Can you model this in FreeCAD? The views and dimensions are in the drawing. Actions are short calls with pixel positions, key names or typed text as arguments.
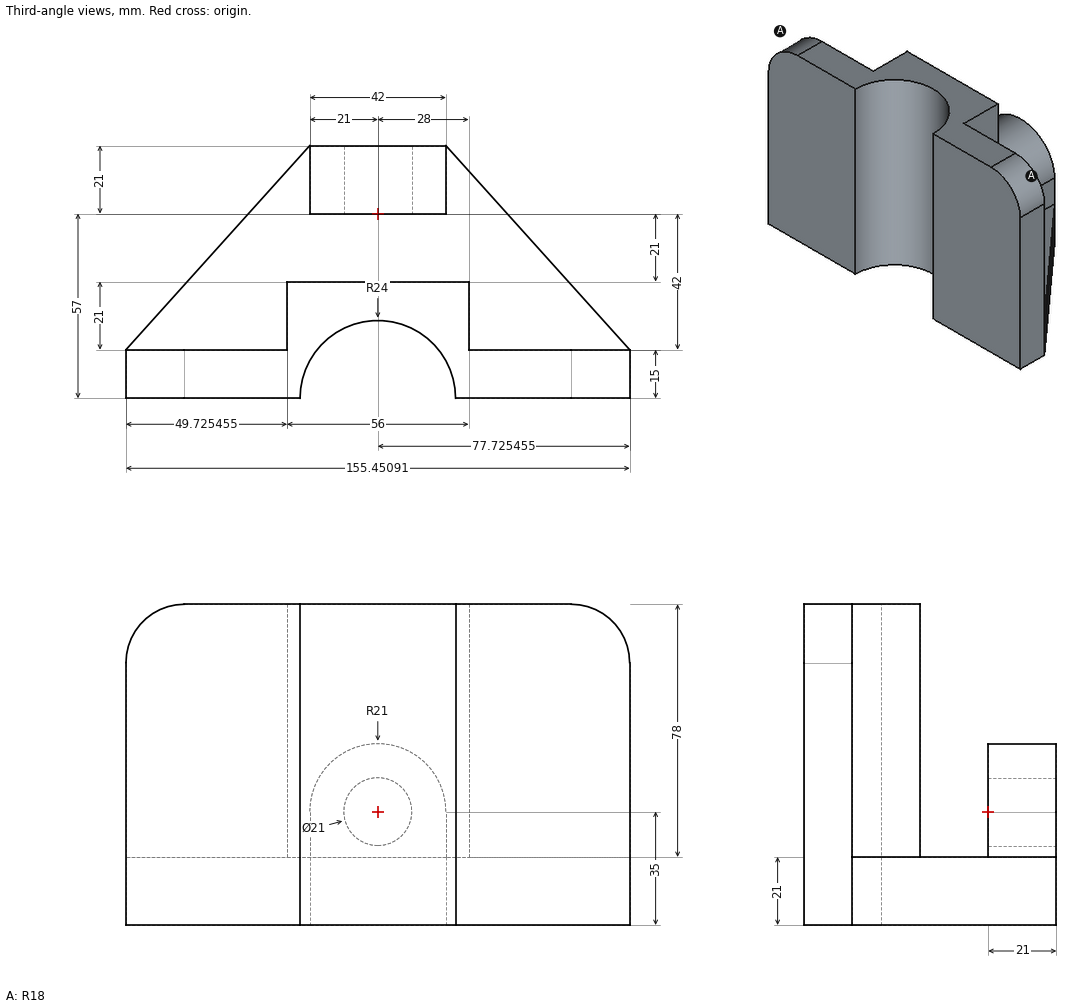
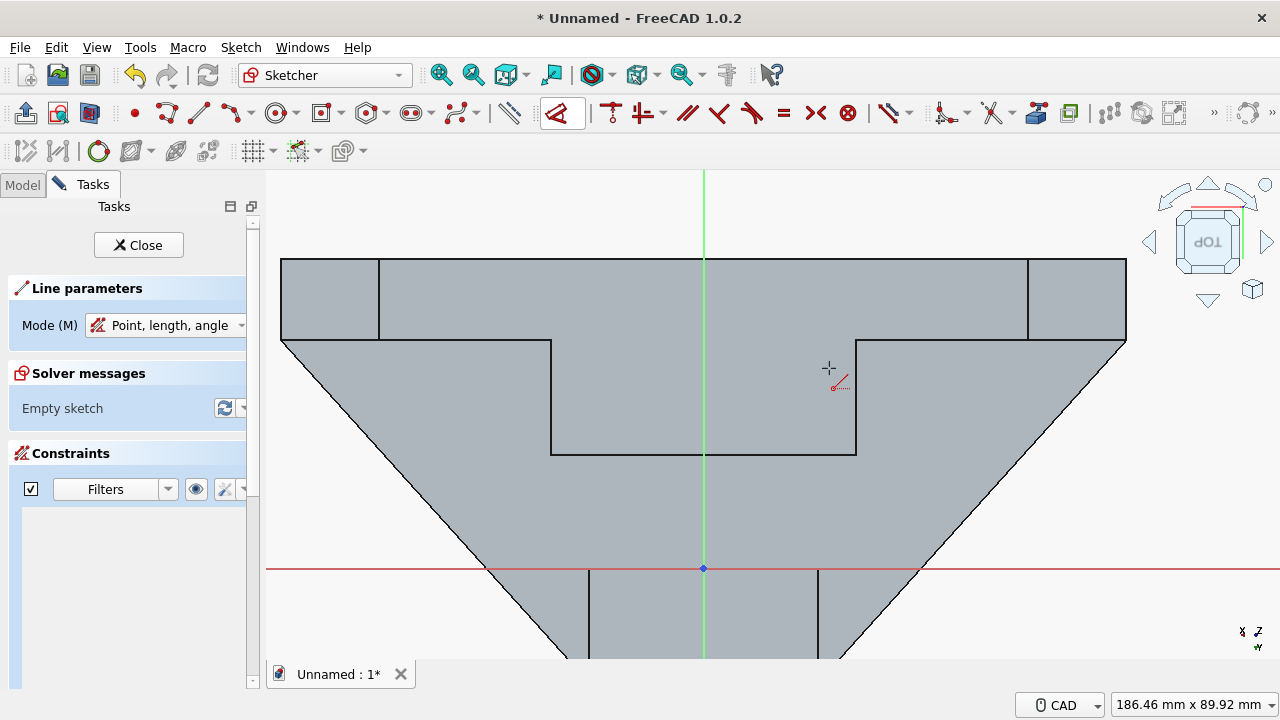
click(834, 259)
click(573, 259)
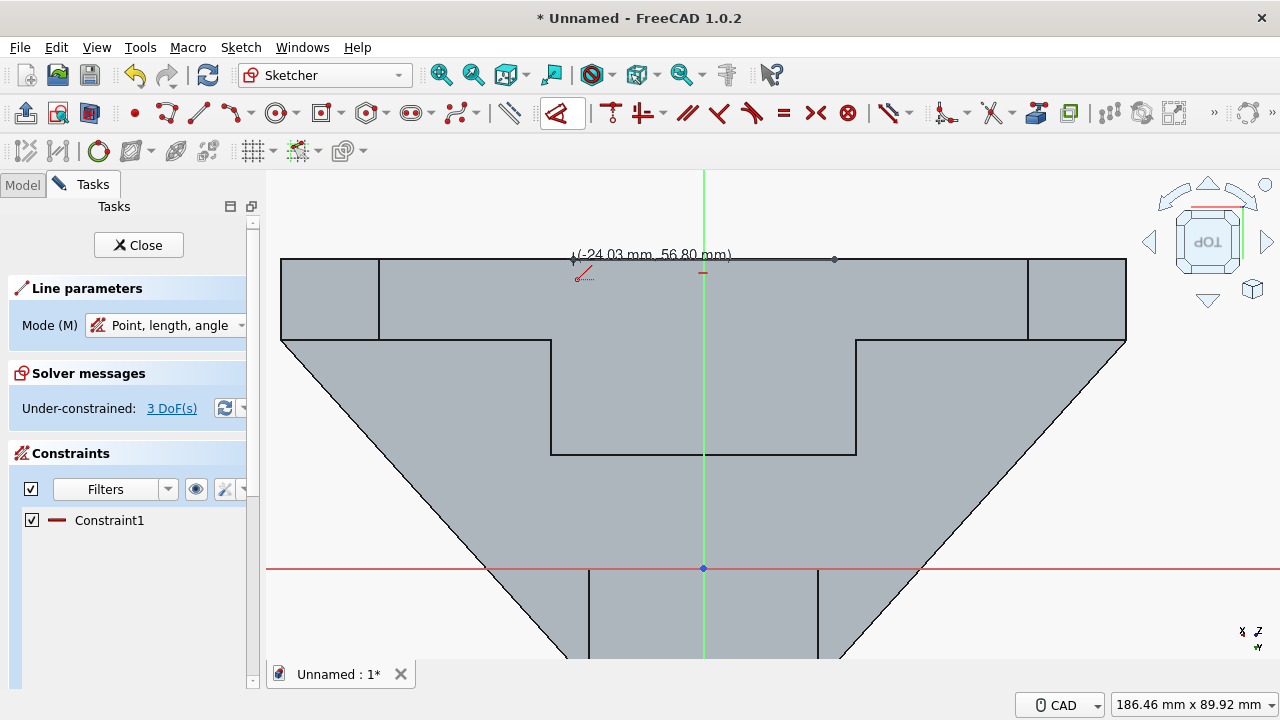
click(232, 114)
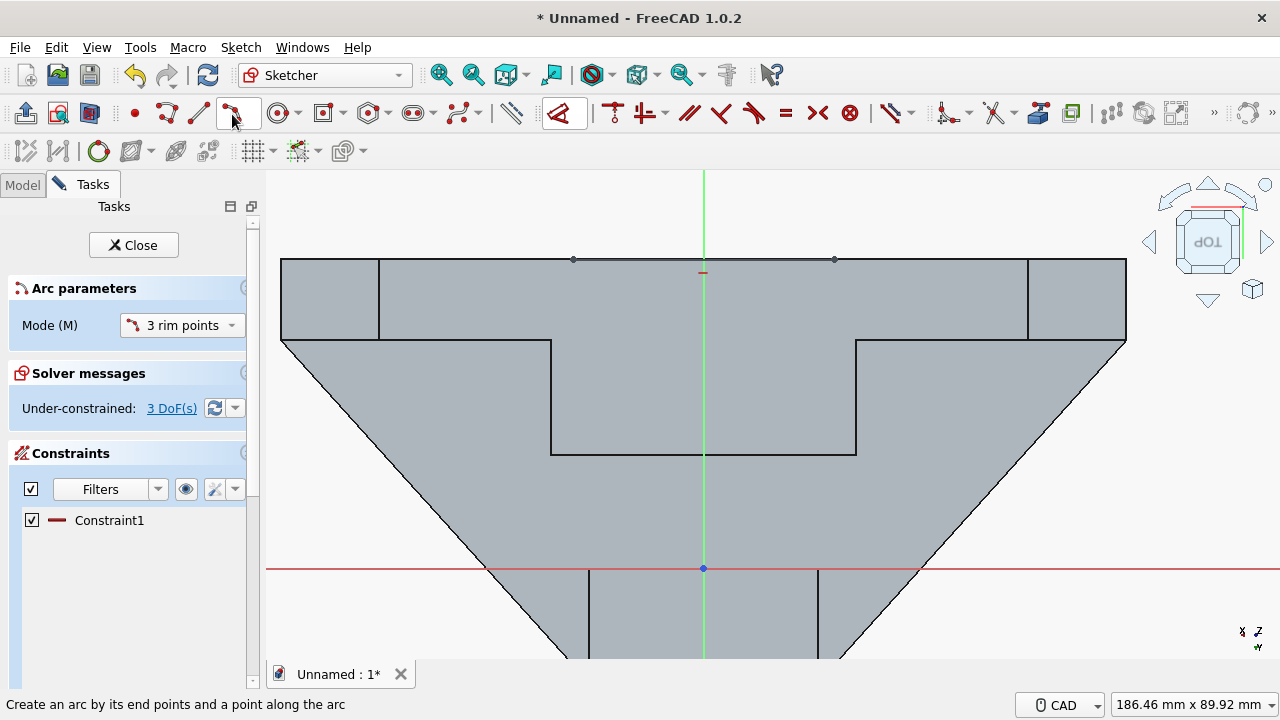
click(573, 260)
click(834, 260)
click(663, 383)
key(Escape)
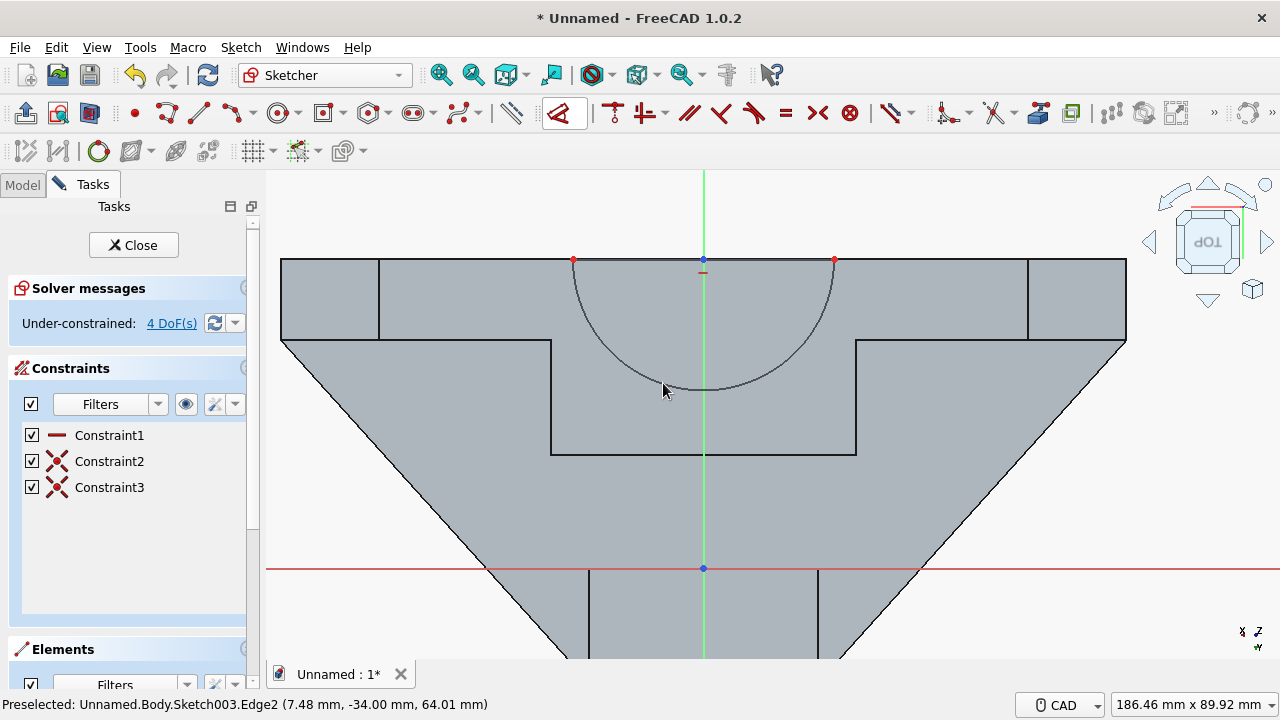
click(704, 260)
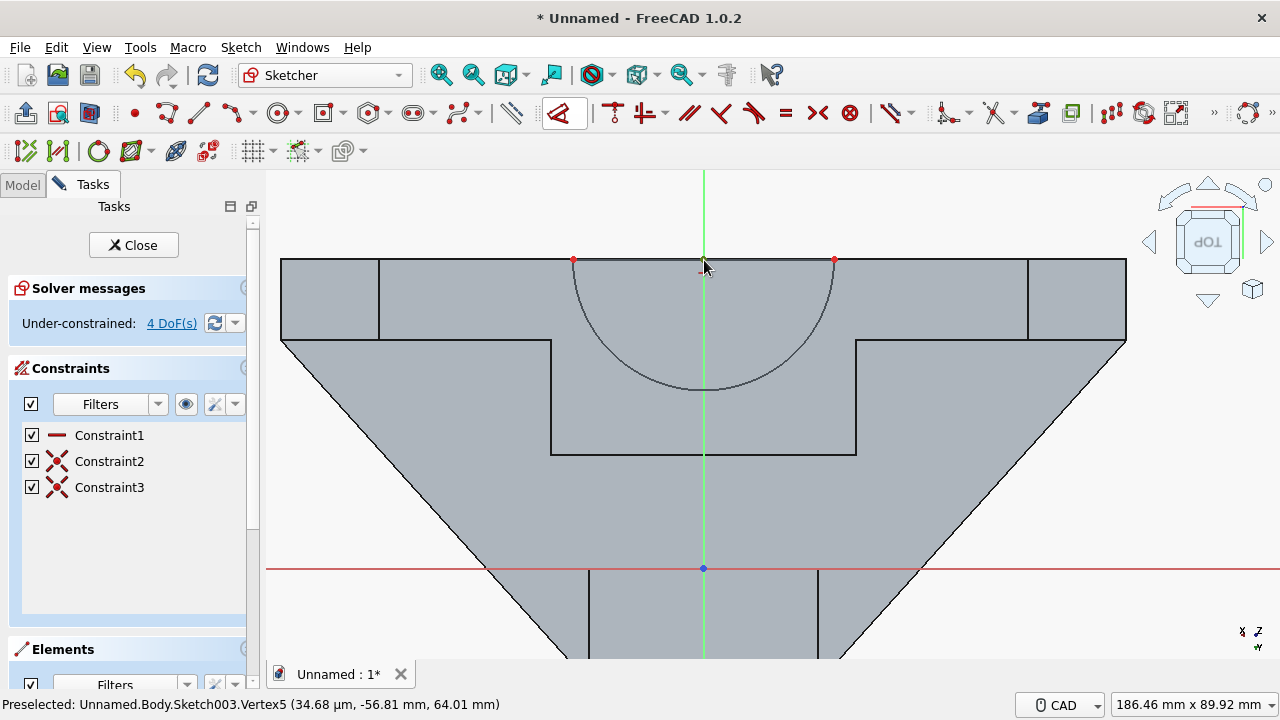
click(704, 600)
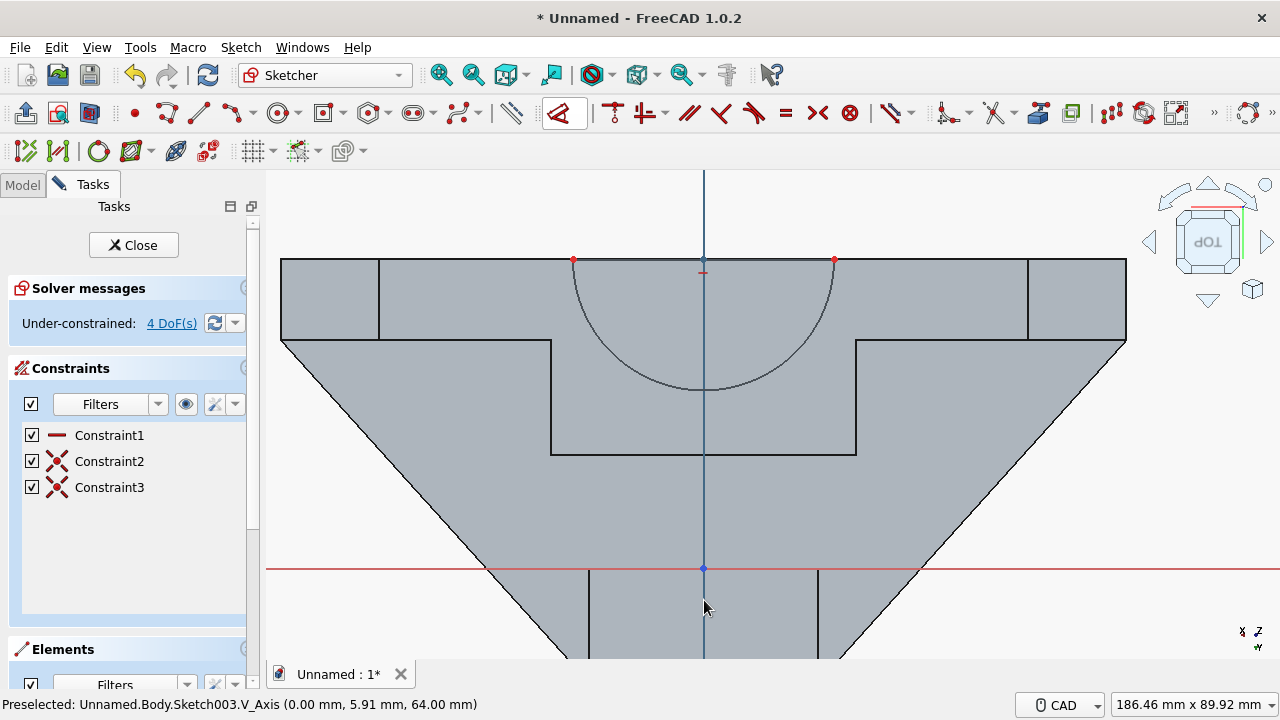
click(614, 114)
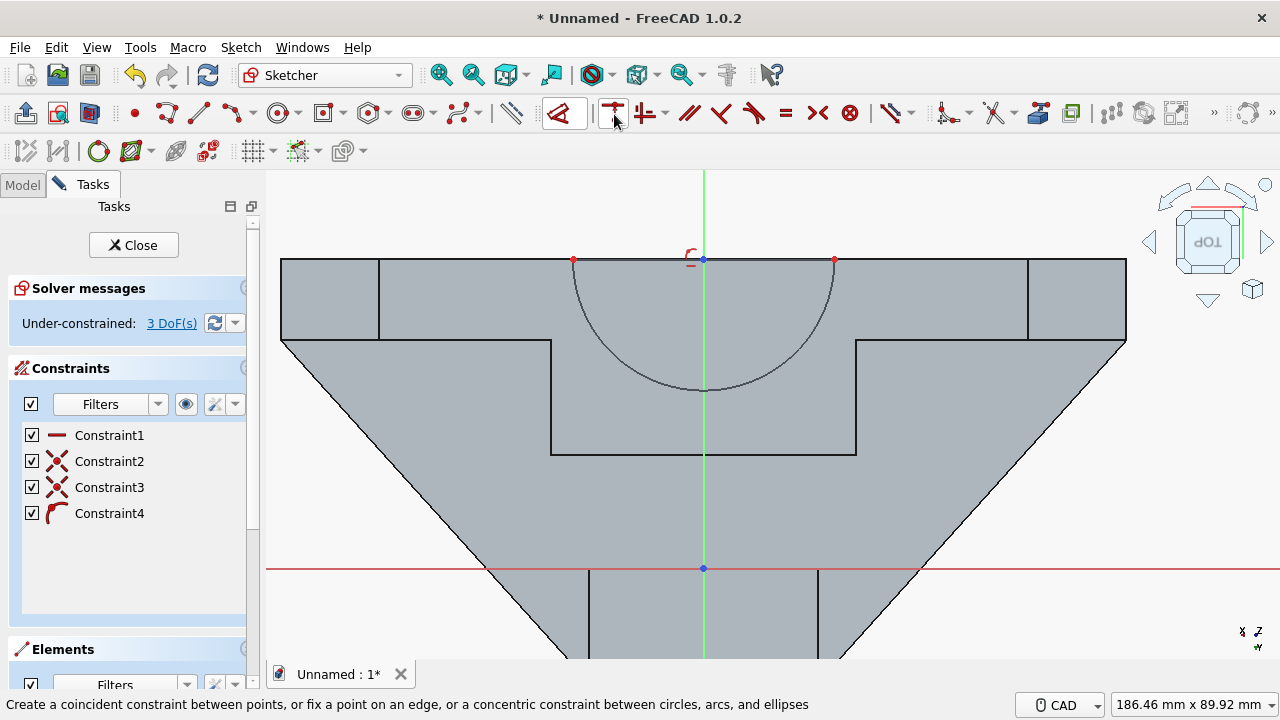
click(627, 366)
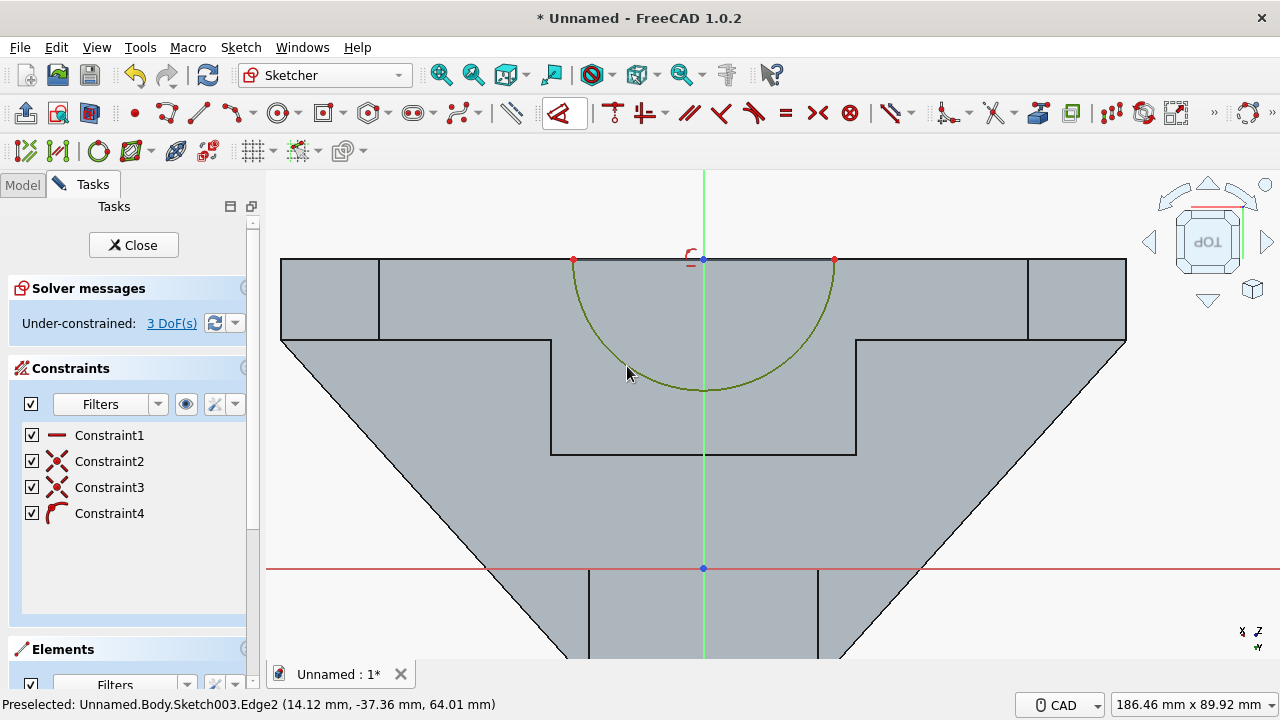
click(582, 114)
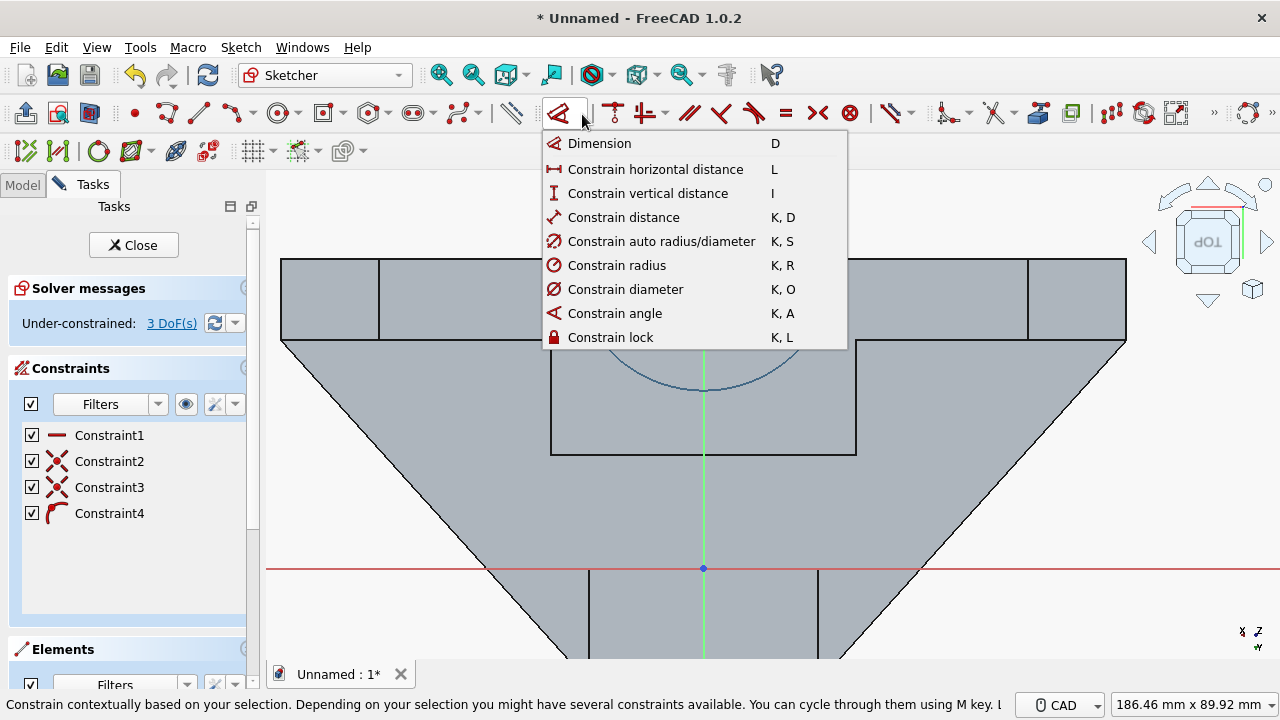
click(695, 265)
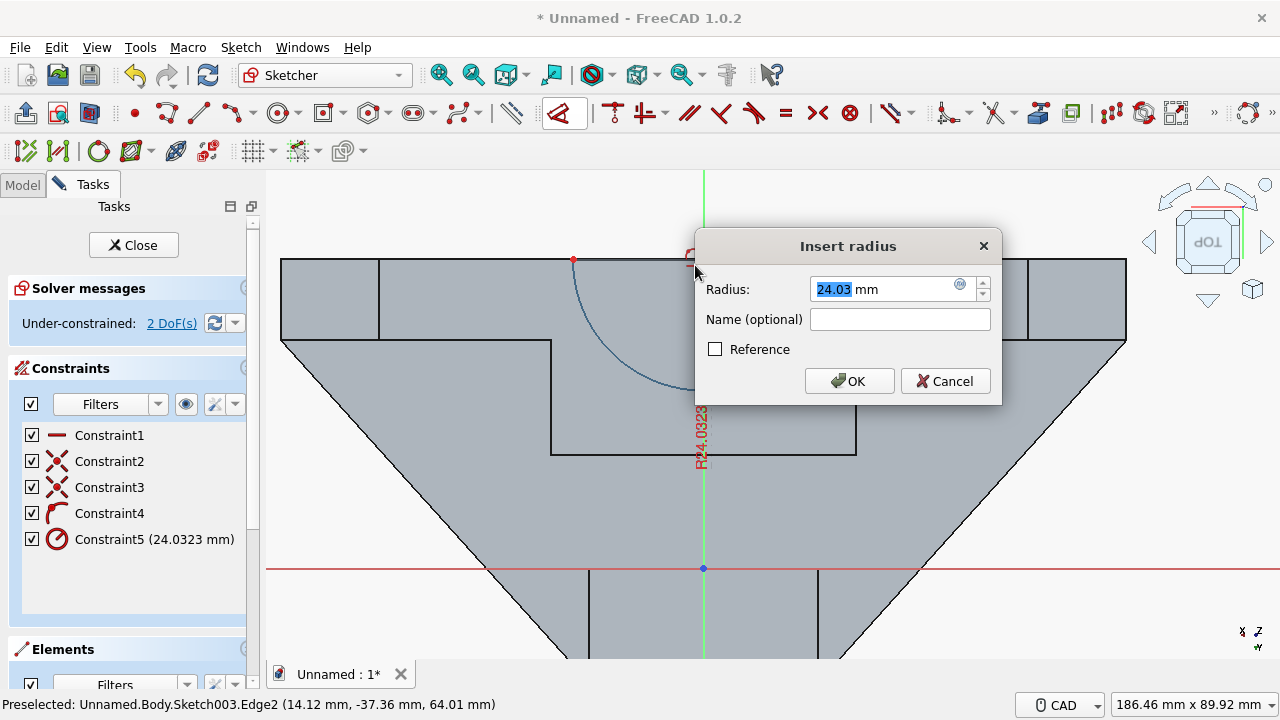
text(24)
key(Return)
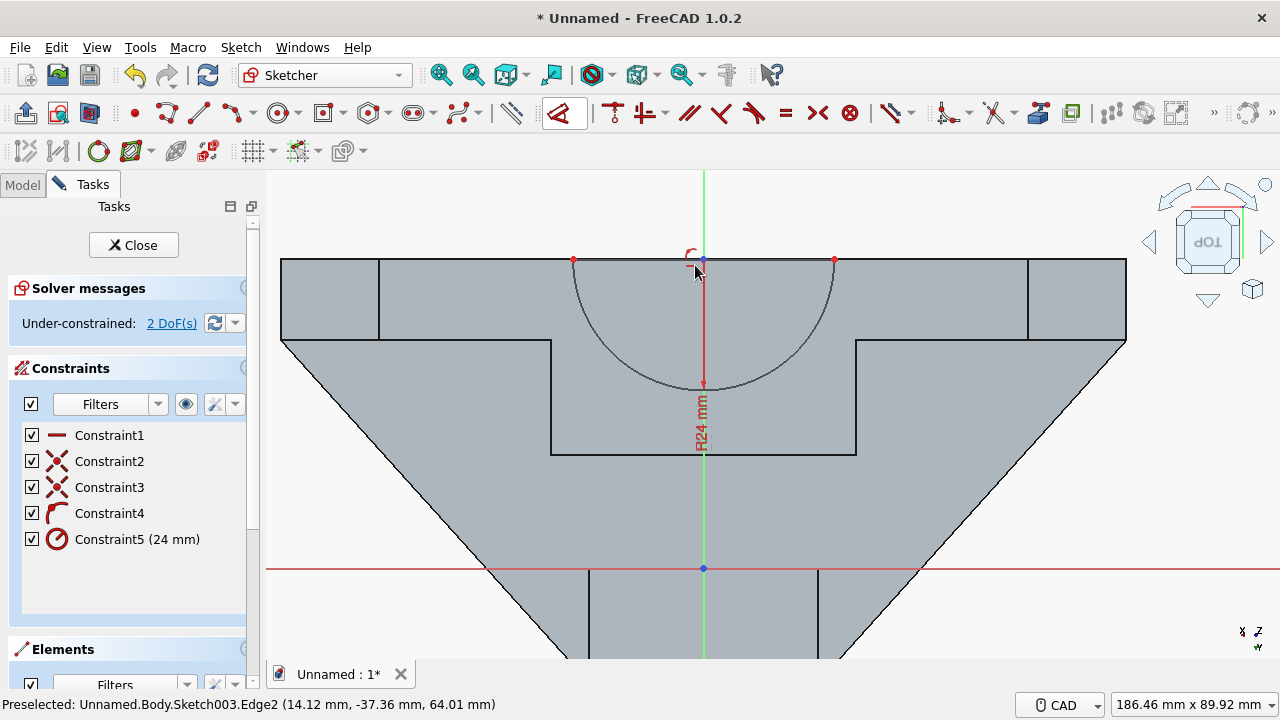
click(834, 260)